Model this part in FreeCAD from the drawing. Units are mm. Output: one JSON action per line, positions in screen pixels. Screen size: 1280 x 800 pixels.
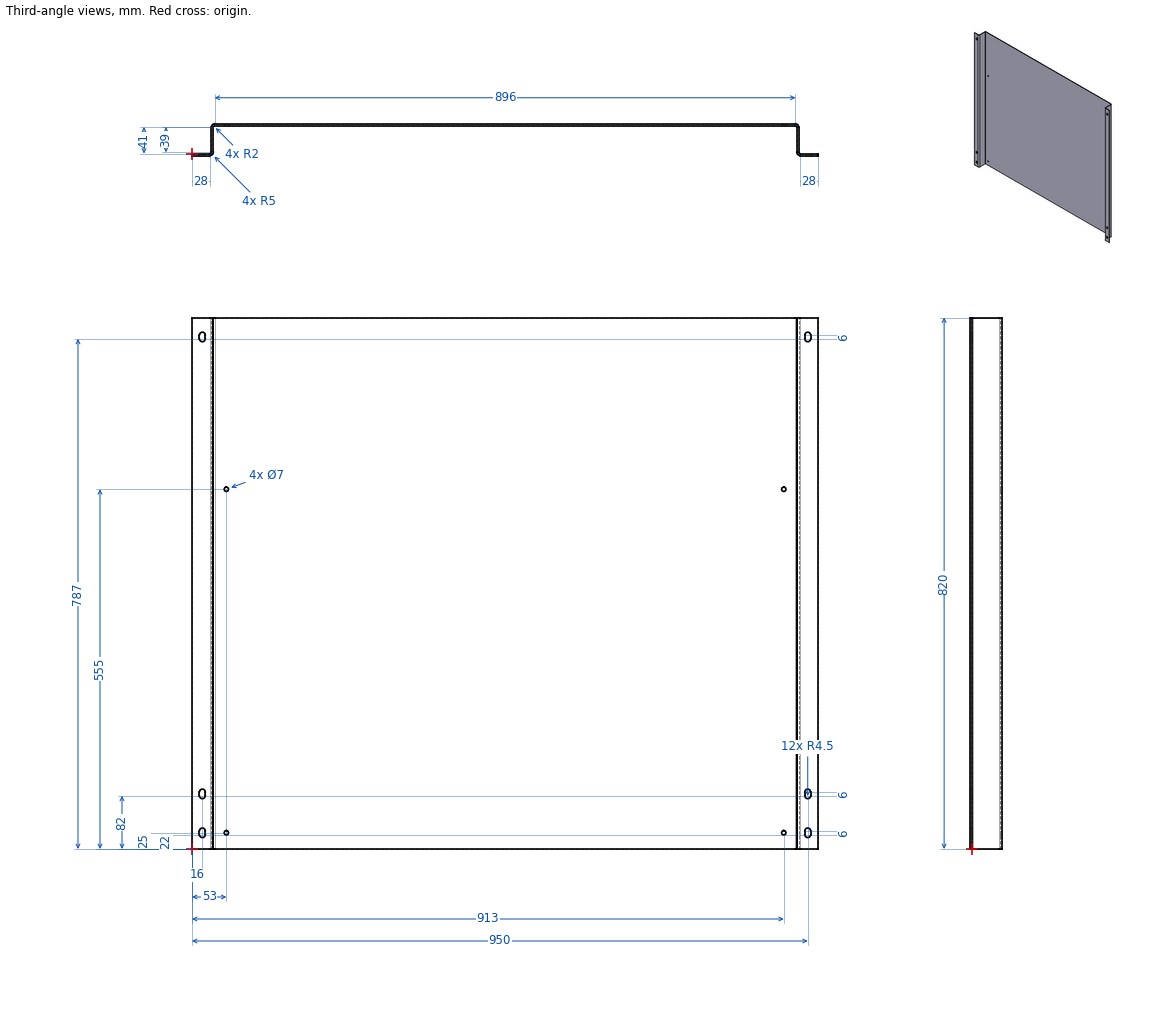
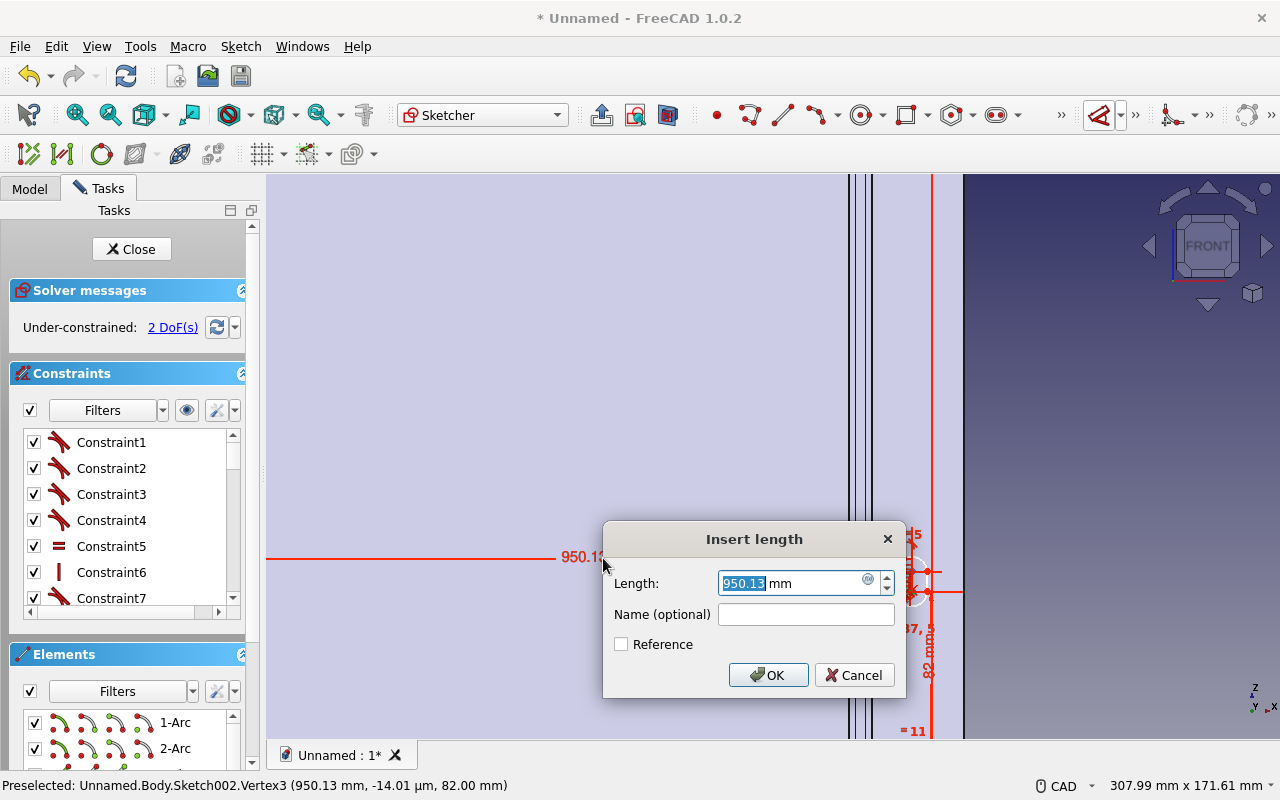
{"action": "type", "text": "950"}
{"action": "key", "text": "Return"}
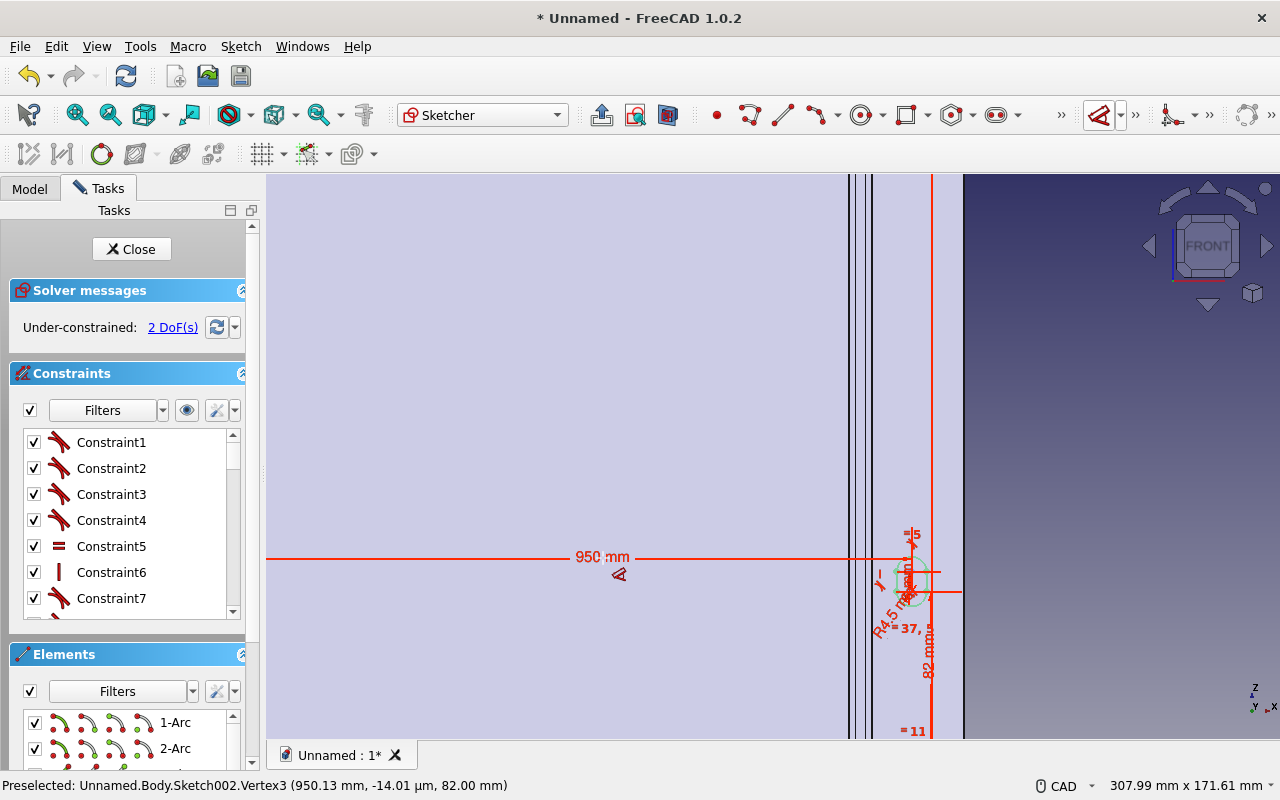
{"action": "scroll", "coordinate": [916, 599], "scroll_direction": "down", "scroll_amount": 10}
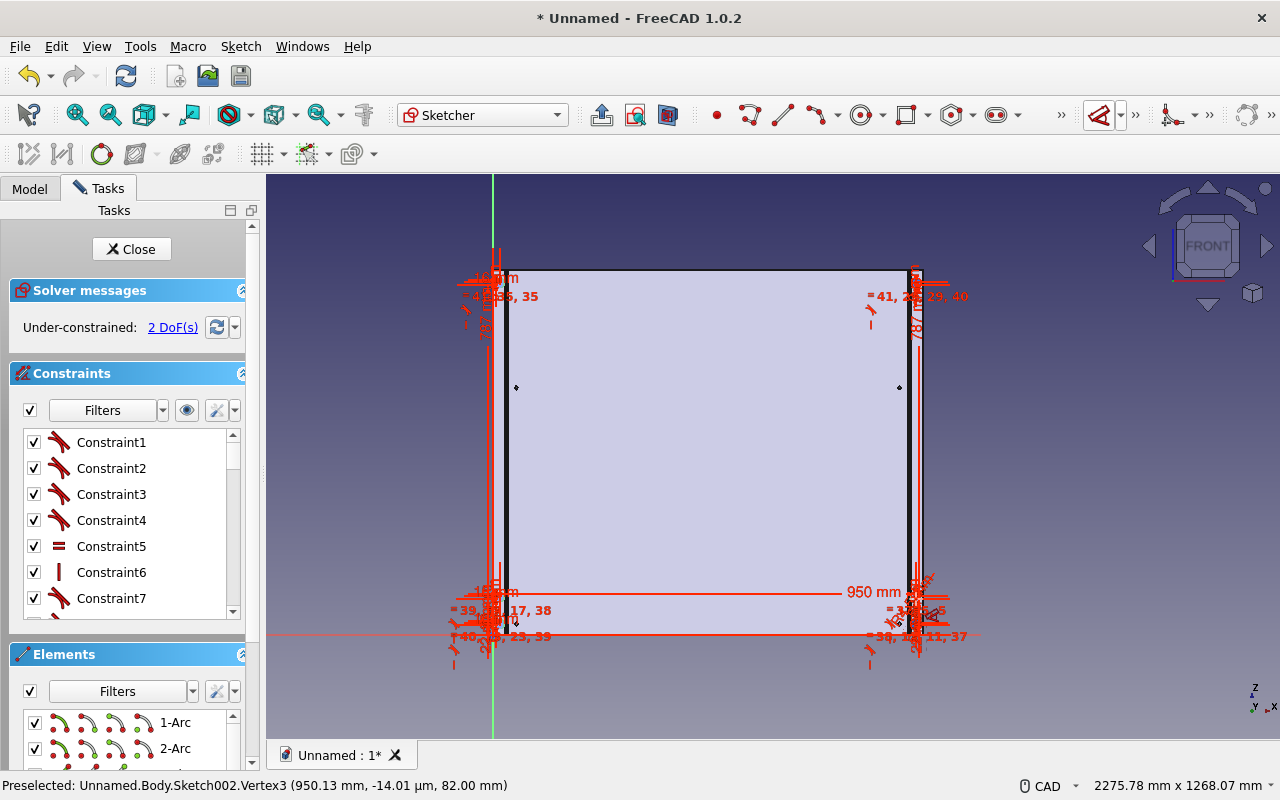
{"action": "scroll", "coordinate": [916, 625], "scroll_direction": "up", "scroll_amount": 10}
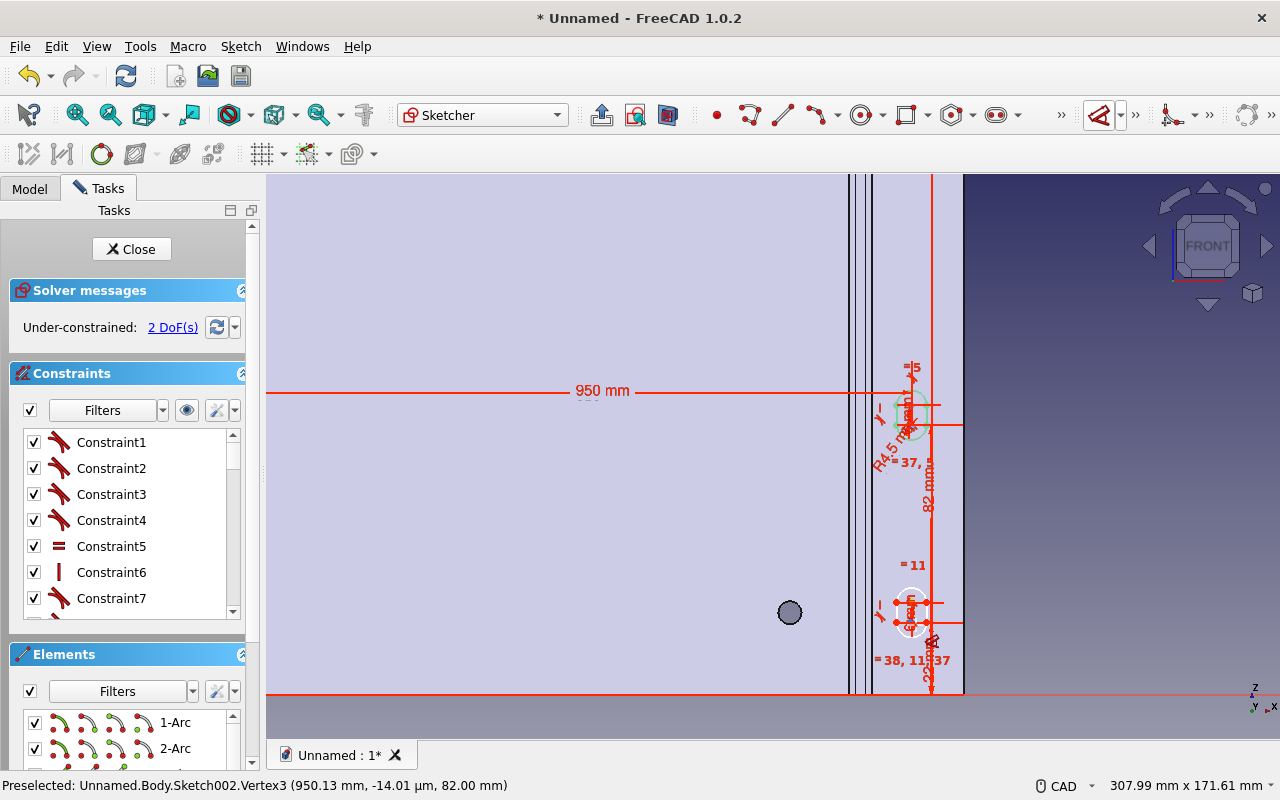
{"action": "left_click", "coordinate": [912, 623]}
{"action": "left_click", "coordinate": [603, 589]}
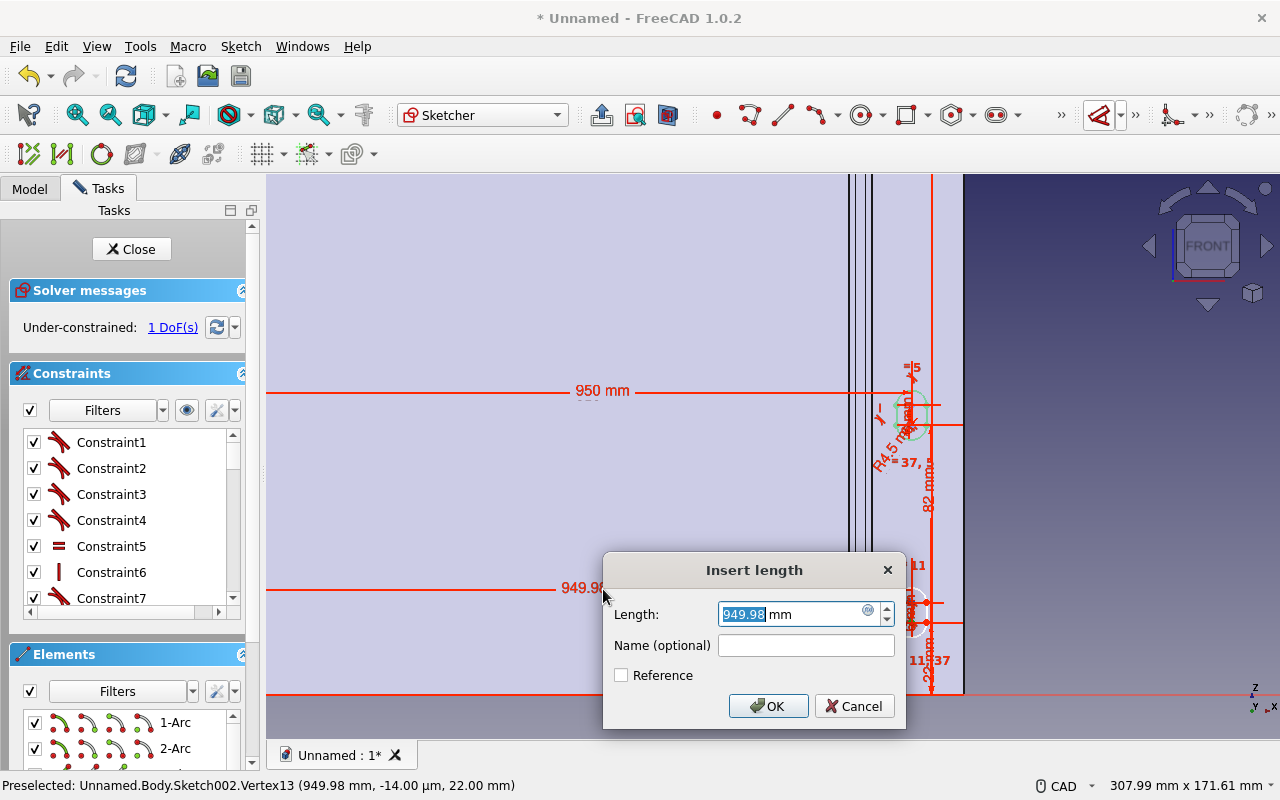
{"action": "type", "text": "950"}
{"action": "key", "text": "Return"}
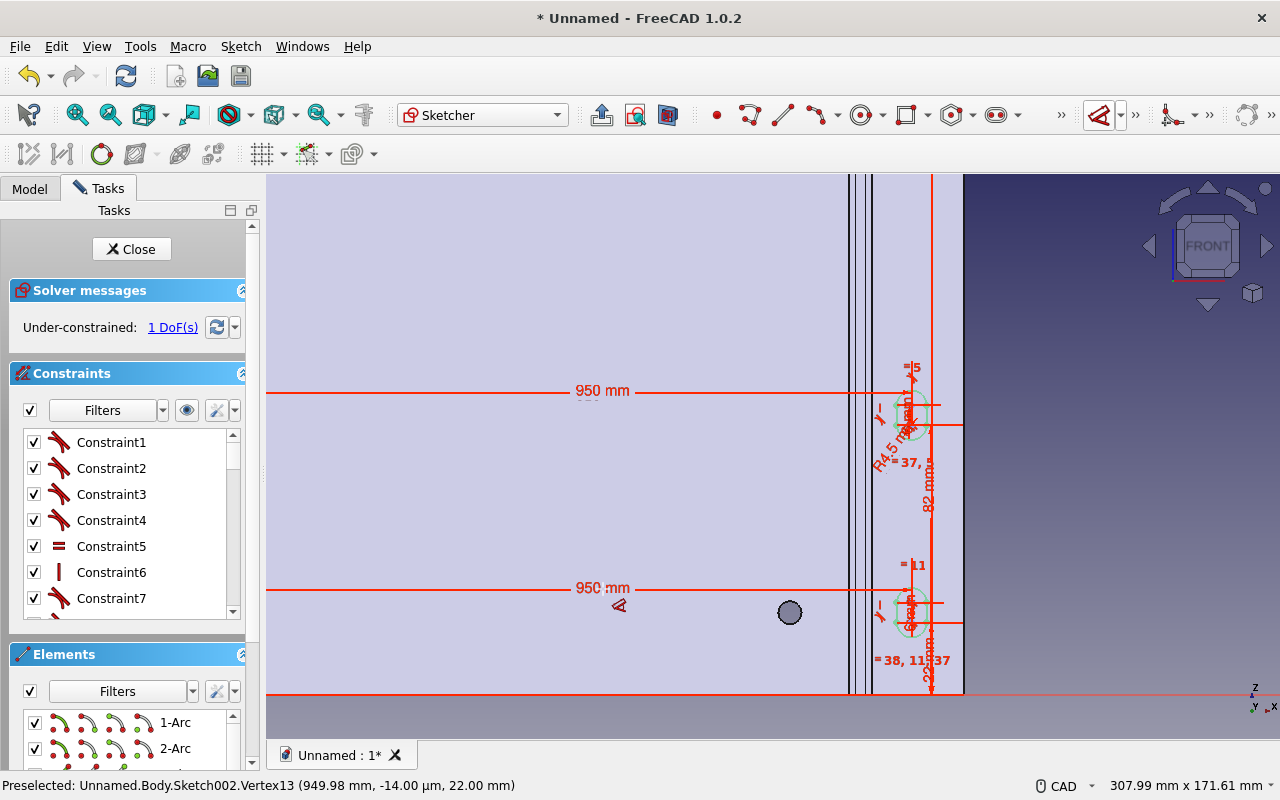
{"action": "scroll", "coordinate": [916, 625], "scroll_direction": "down", "scroll_amount": 10}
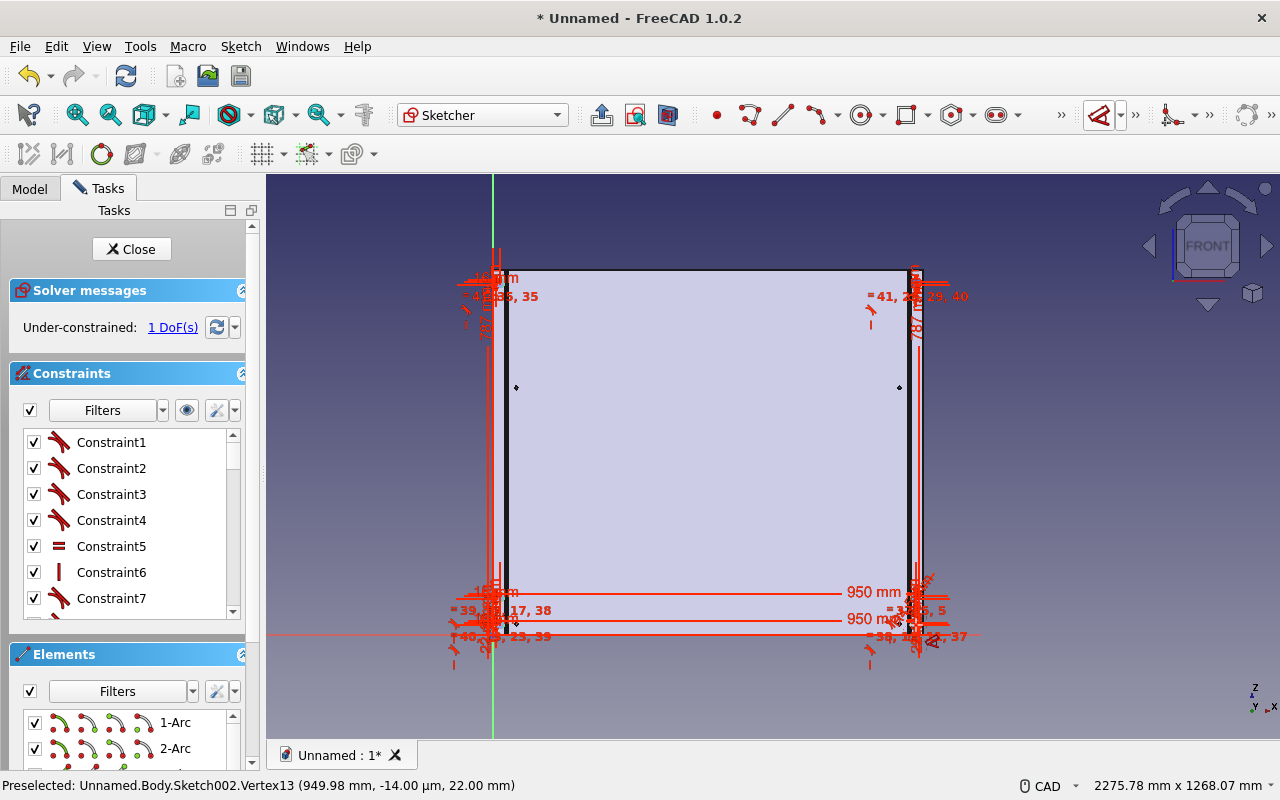
{"action": "scroll", "coordinate": [916, 285], "scroll_direction": "up", "scroll_amount": 10}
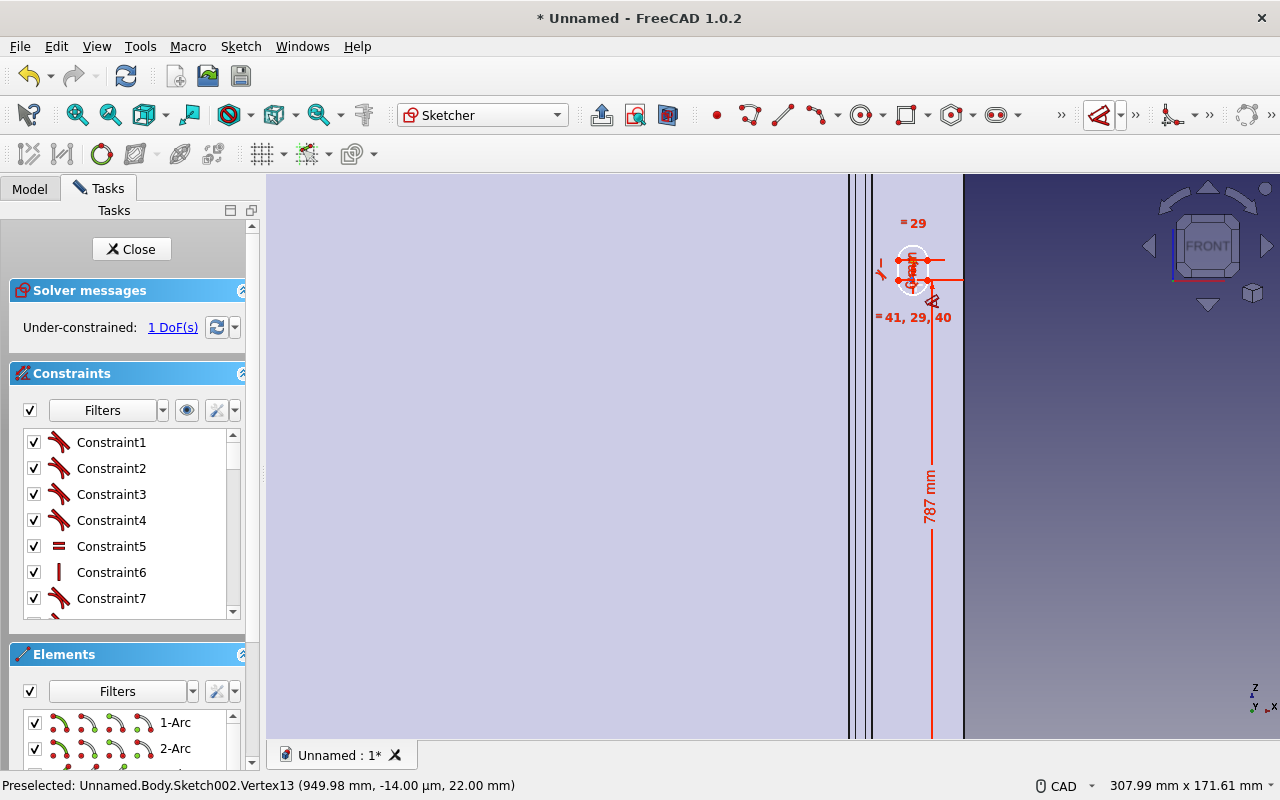
{"action": "left_click", "coordinate": [913, 280]}
{"action": "left_click", "coordinate": [603, 246]}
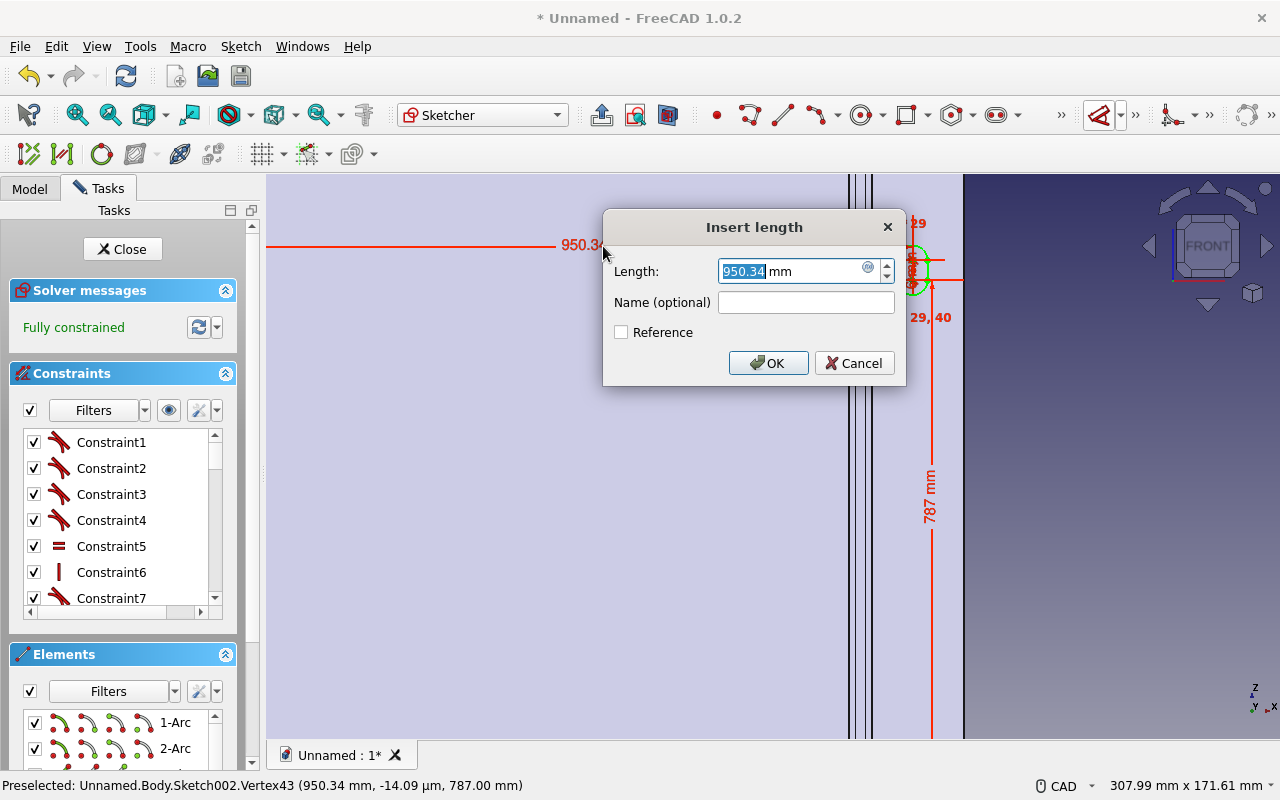
{"action": "type", "text": "950"}
{"action": "key", "text": "Return"}
{"action": "key", "text": "Escape"}